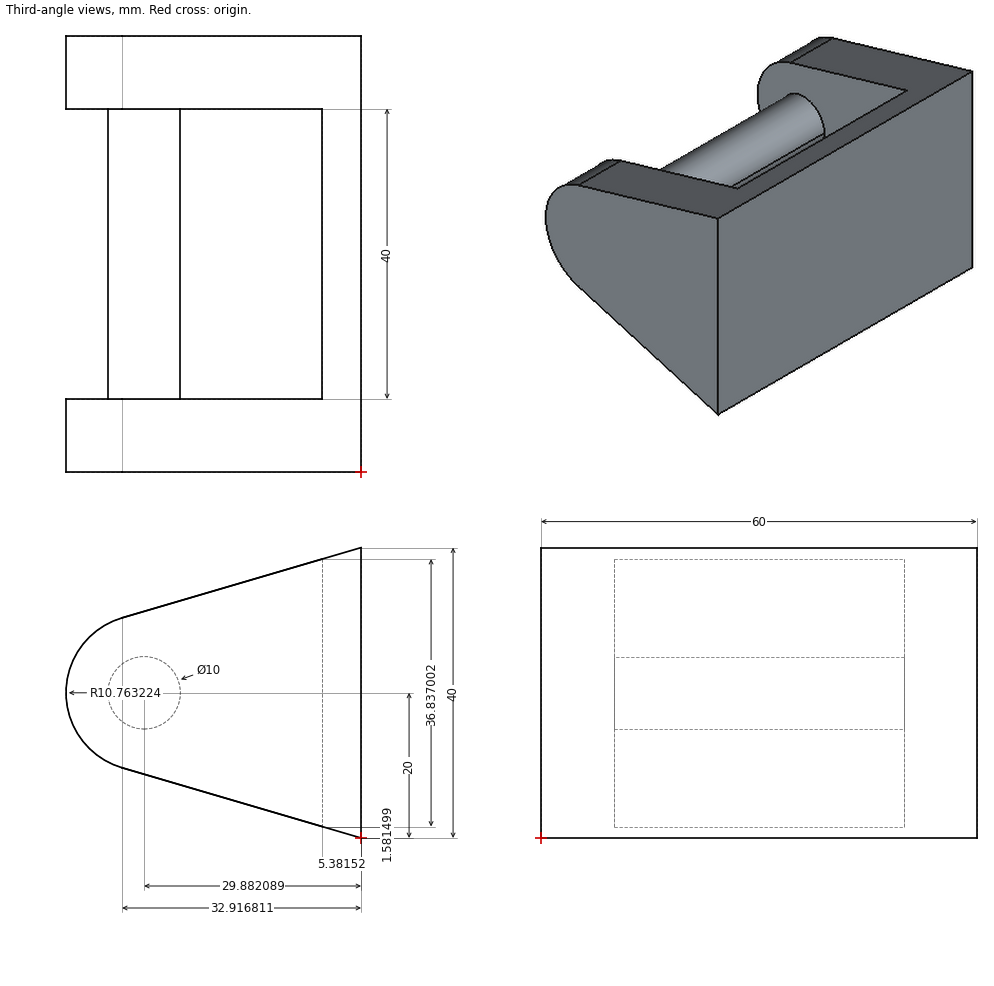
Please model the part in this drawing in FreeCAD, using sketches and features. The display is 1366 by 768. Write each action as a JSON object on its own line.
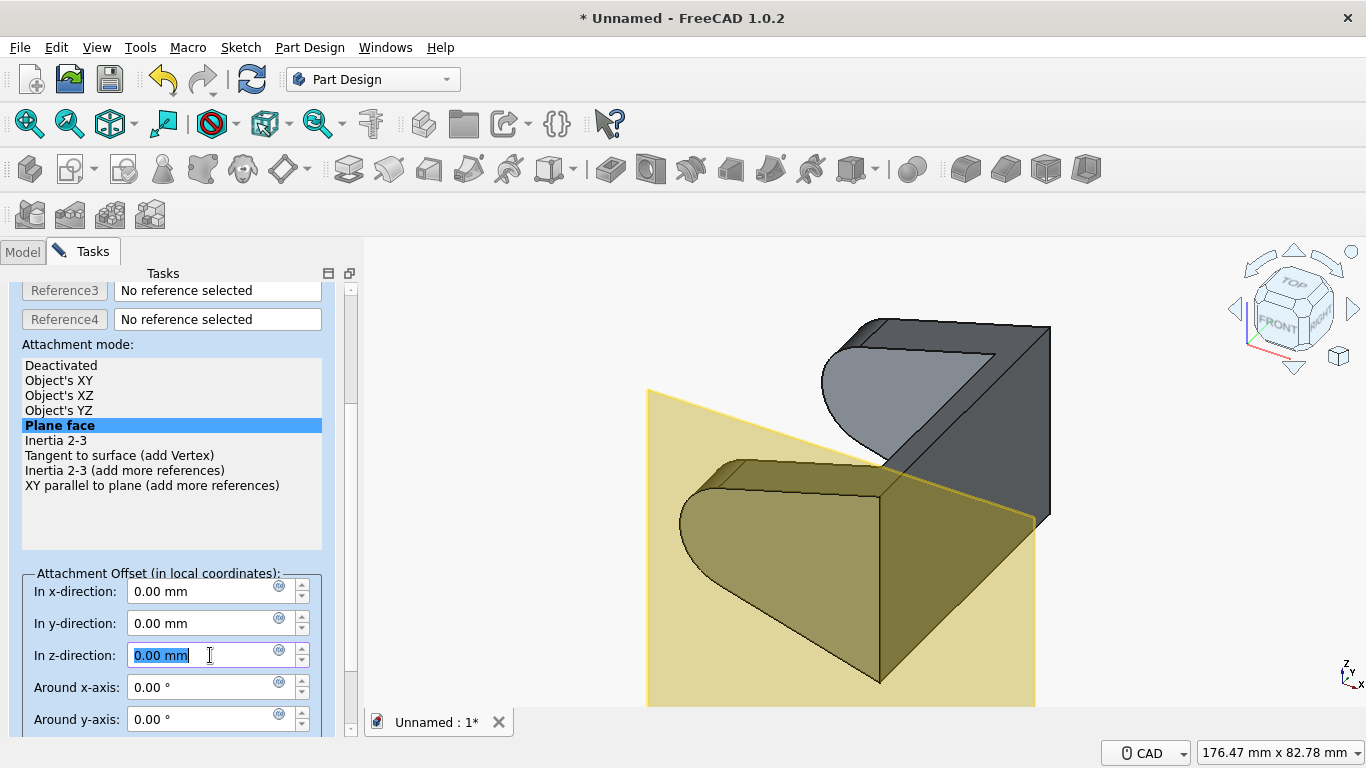
{"action": "type", "text": "-10"}
{"action": "key", "text": "Tab"}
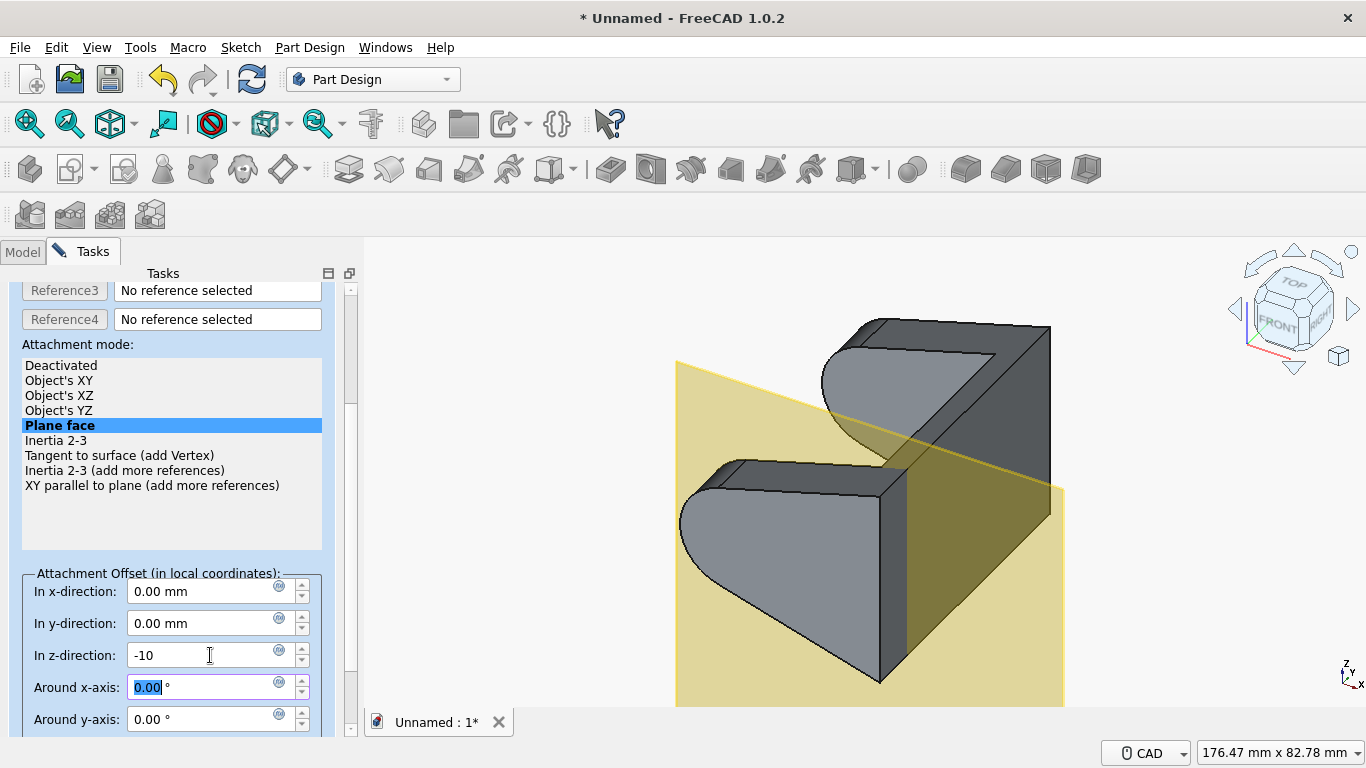
{"action": "scroll", "coordinate": [351, 510], "scroll_direction": "up", "scroll_amount": 4}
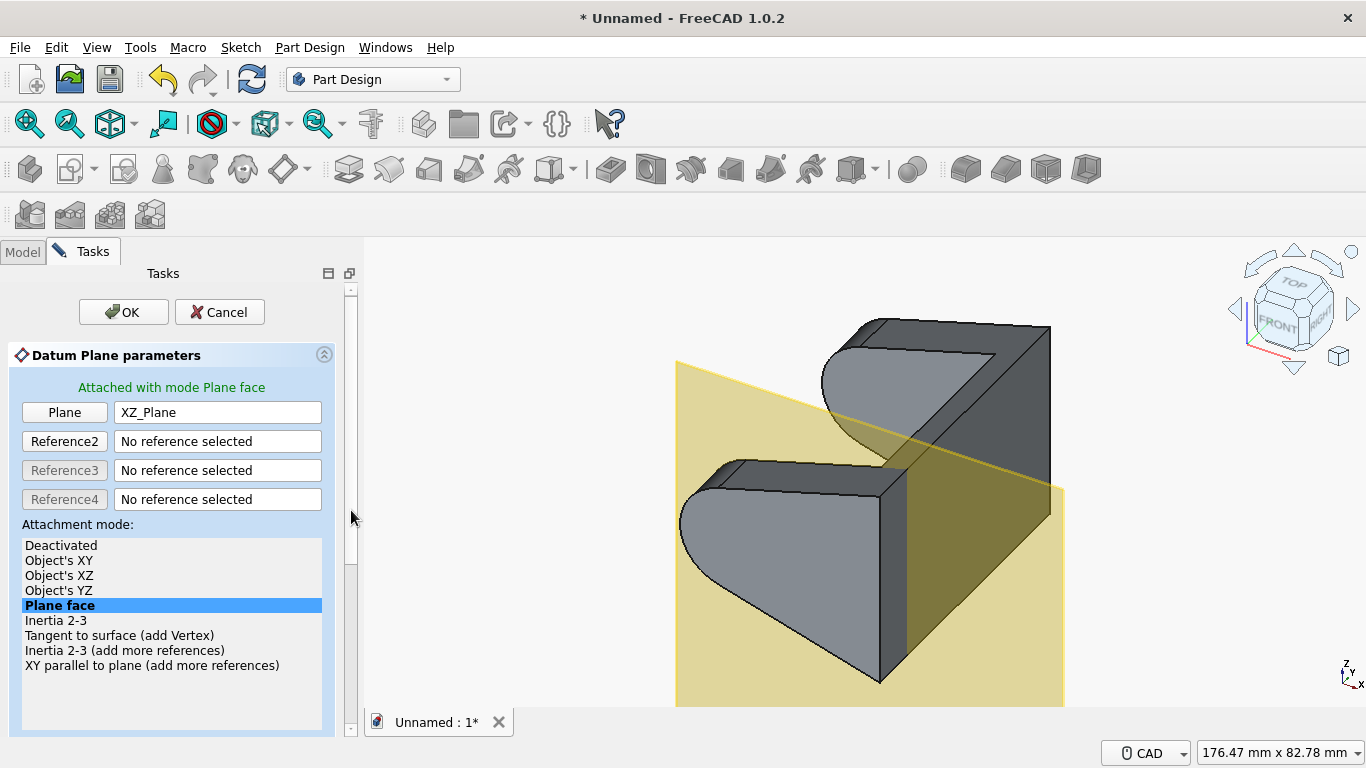
{"action": "left_click", "coordinate": [124, 312]}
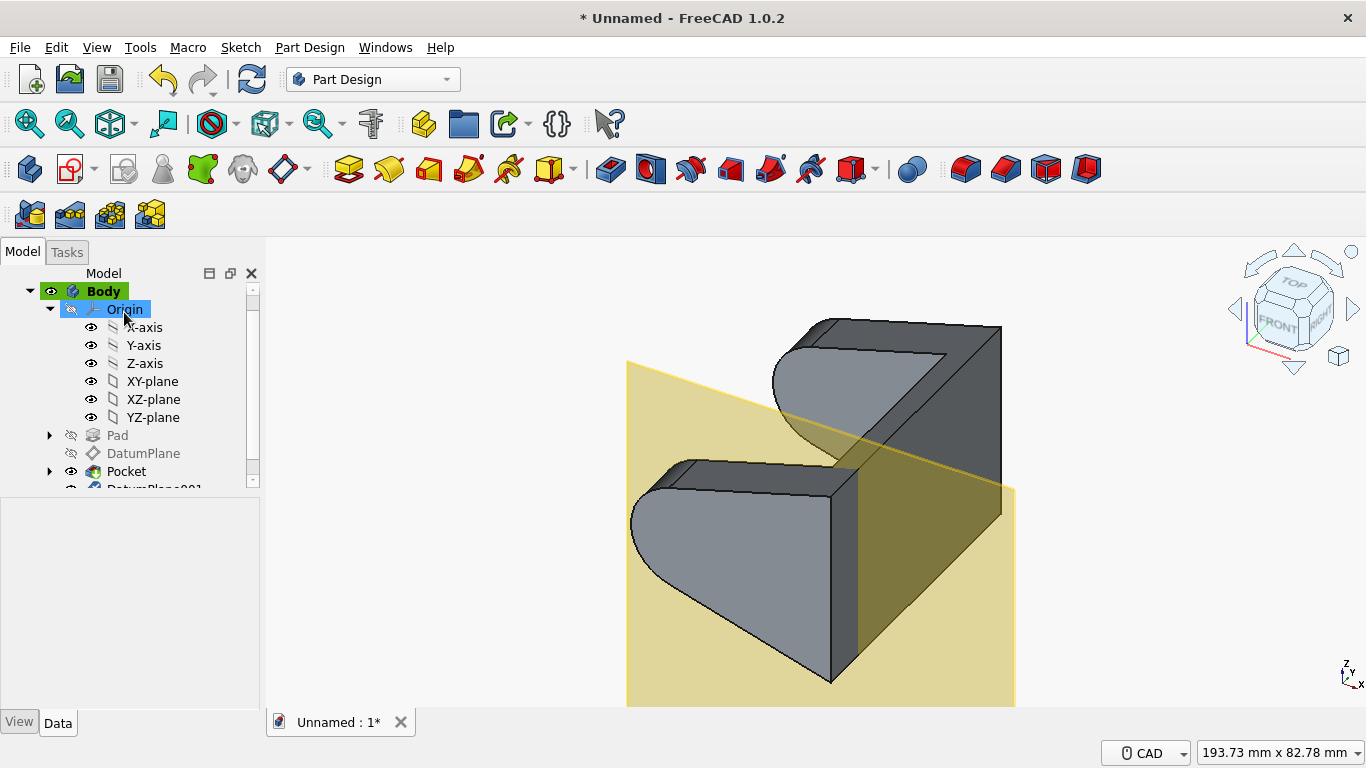
{"action": "scroll", "coordinate": [120, 377], "scroll_direction": "down", "scroll_amount": 3}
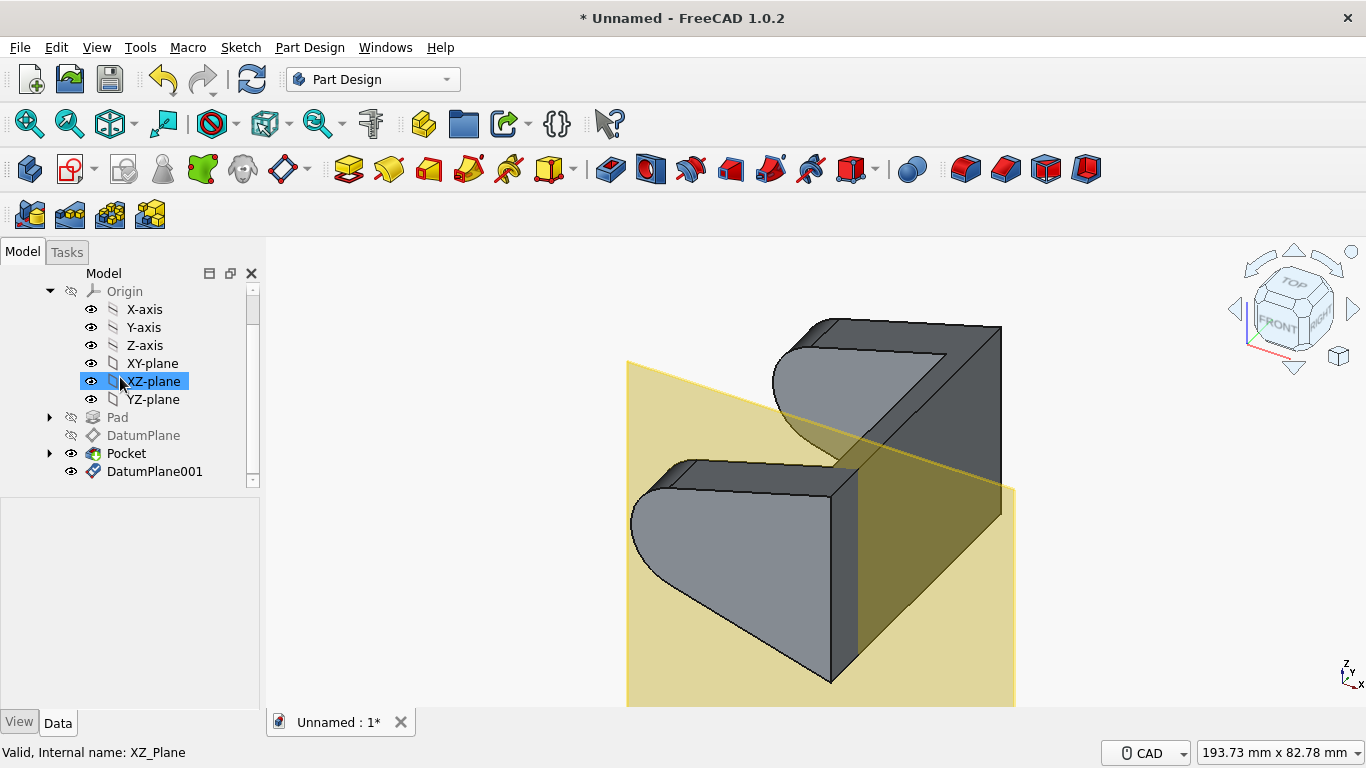
{"action": "left_click", "coordinate": [116, 471]}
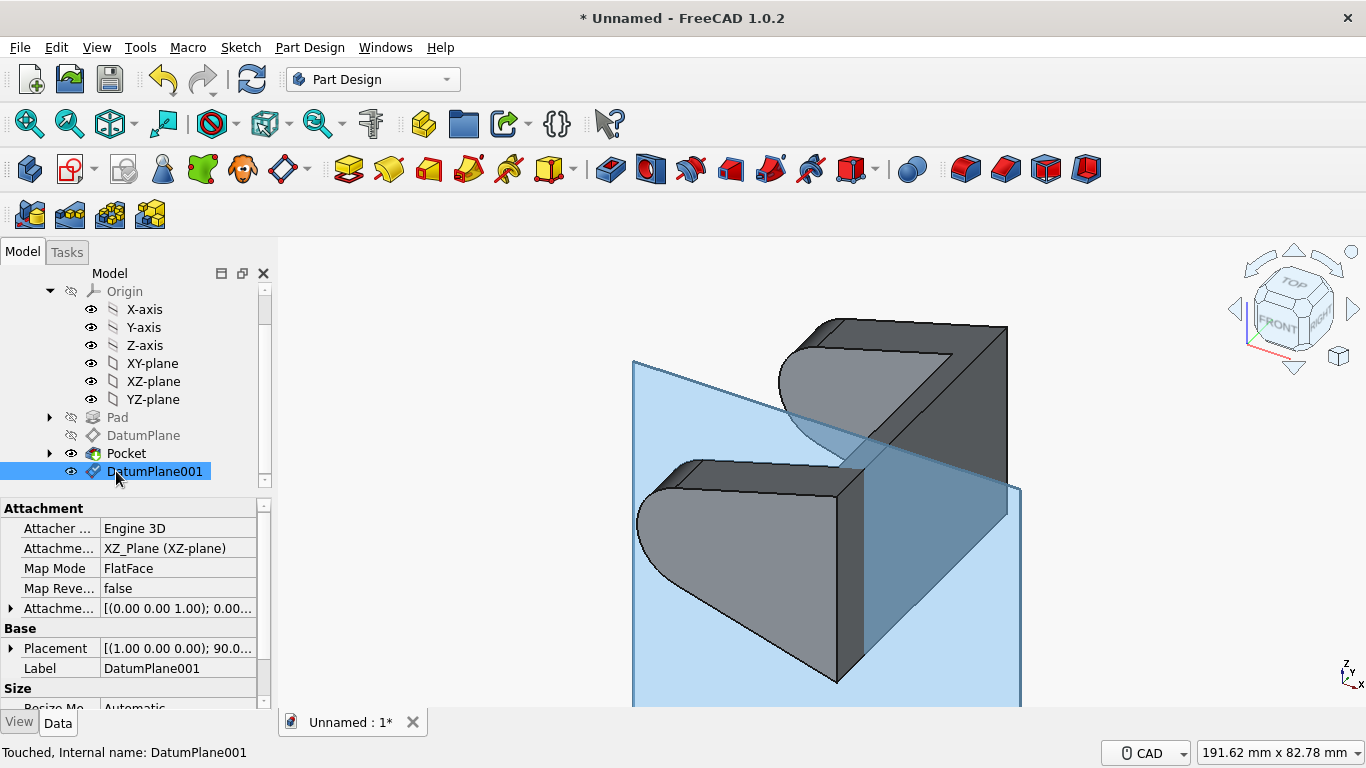
{"action": "left_click", "coordinate": [70, 170]}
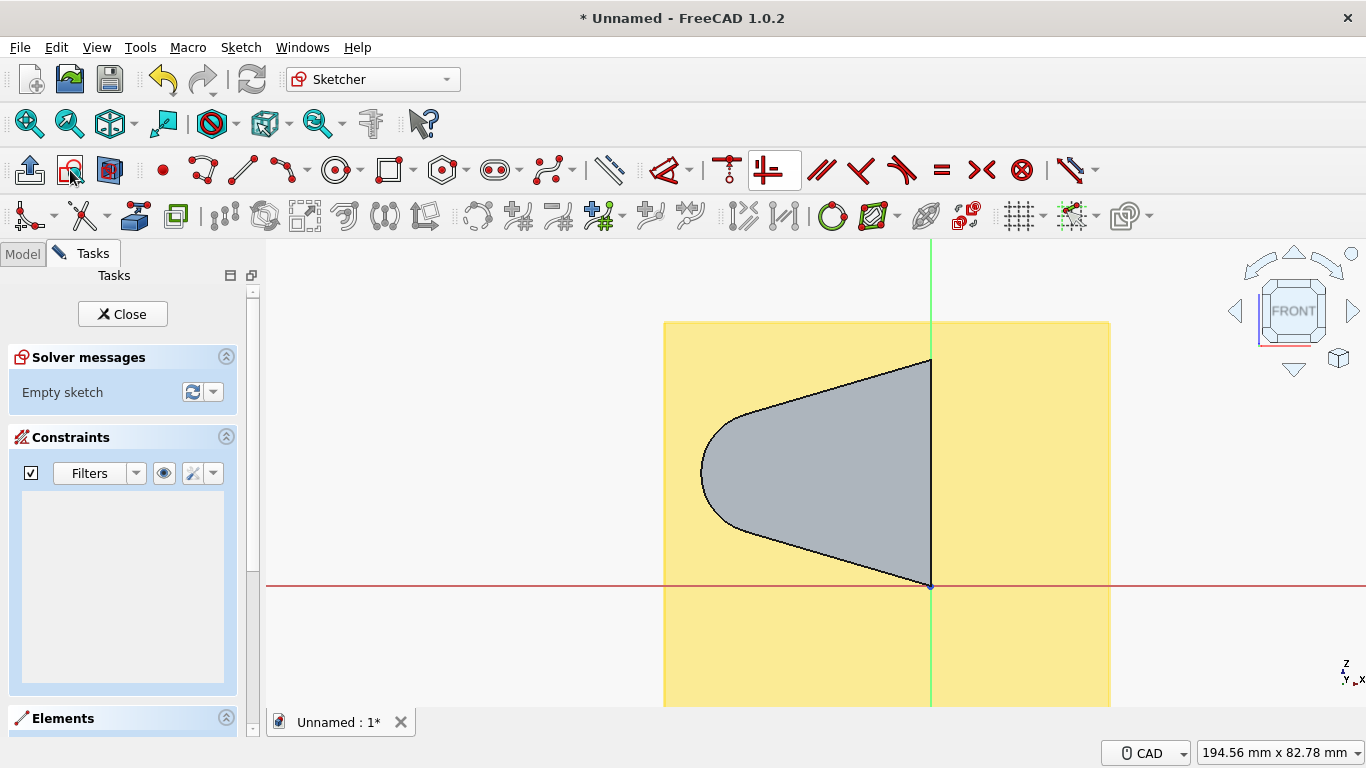
{"action": "left_click", "coordinate": [110, 170]}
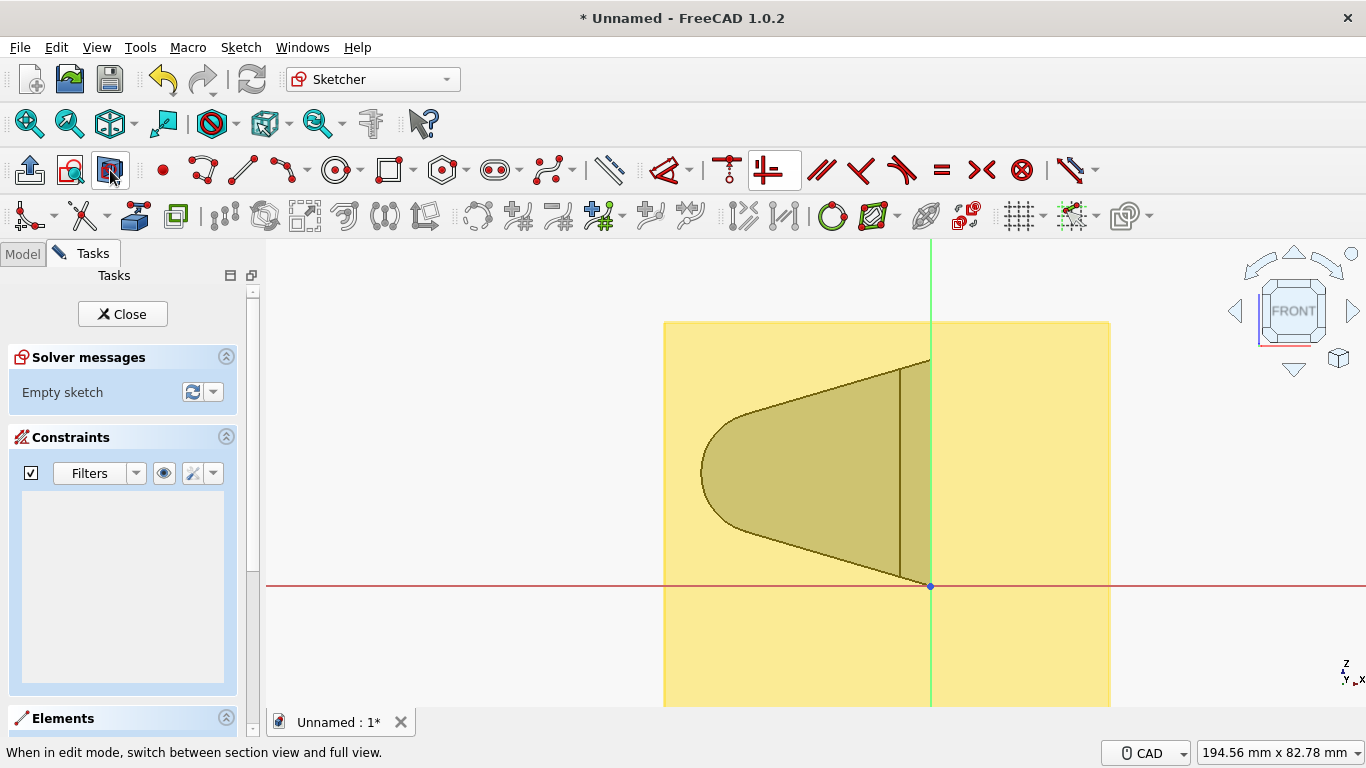
{"action": "scroll", "coordinate": [766, 473], "scroll_direction": "up", "scroll_amount": 8}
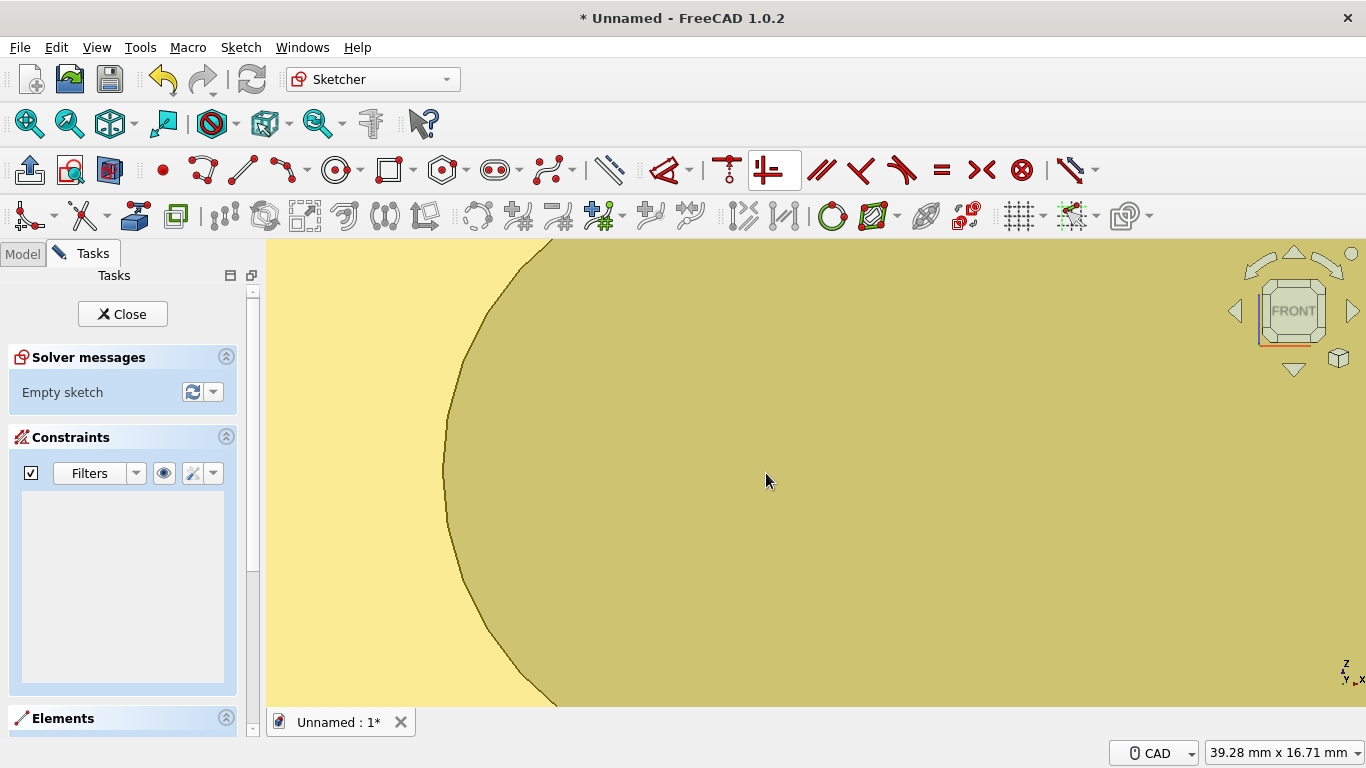
{"action": "left_click", "coordinate": [336, 170]}